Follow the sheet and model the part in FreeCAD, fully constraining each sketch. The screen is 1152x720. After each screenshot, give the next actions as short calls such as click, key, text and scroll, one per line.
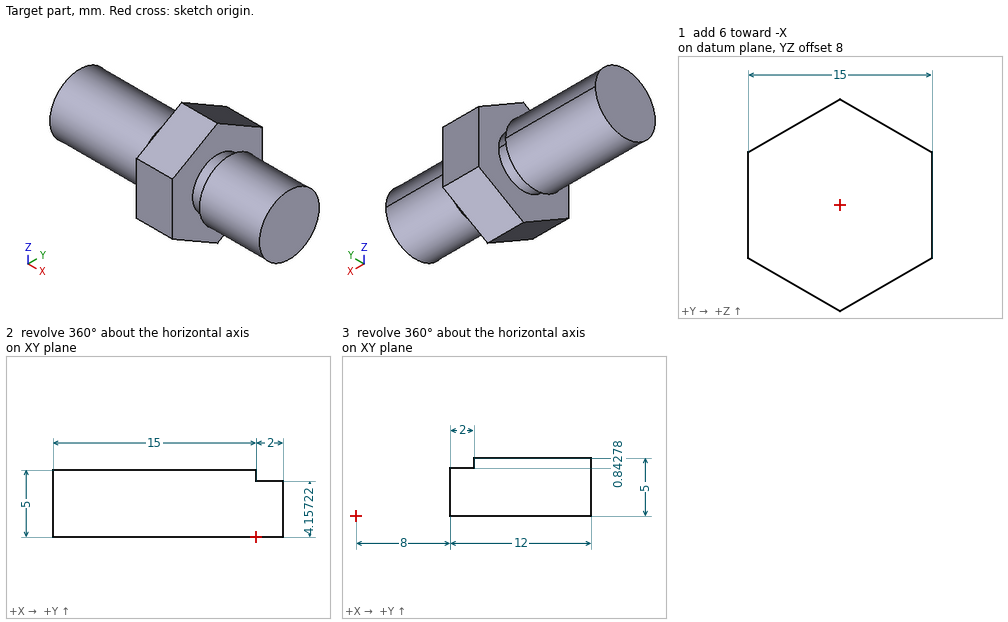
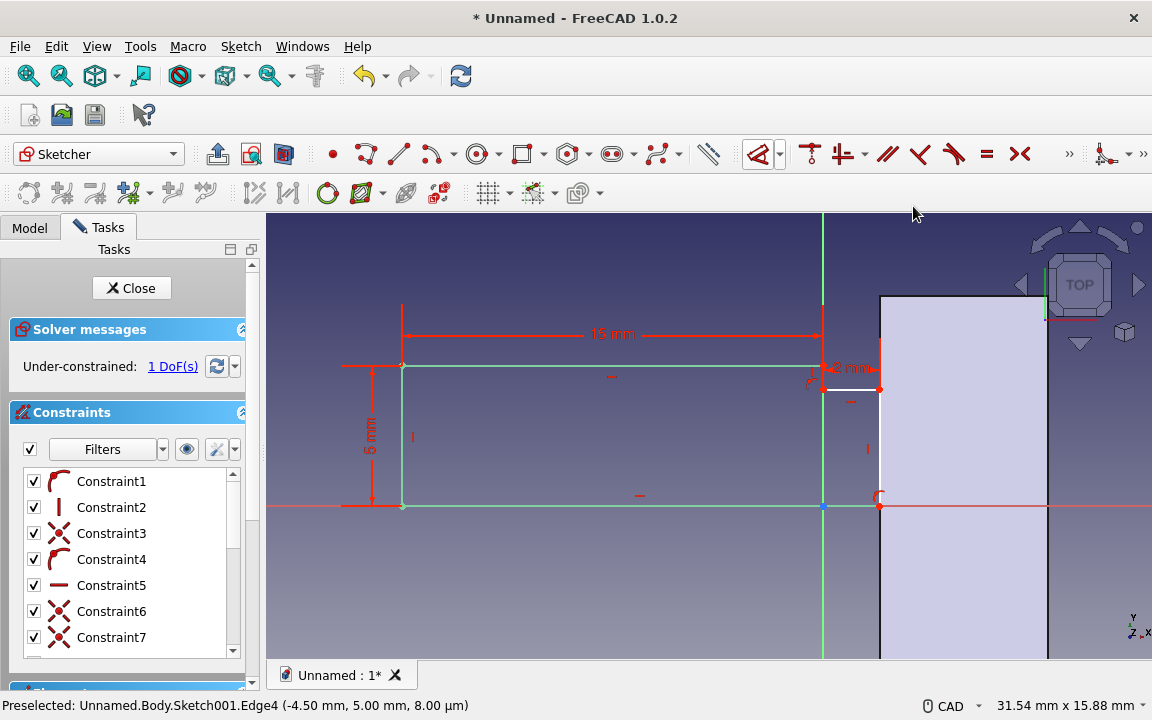
click(880, 471)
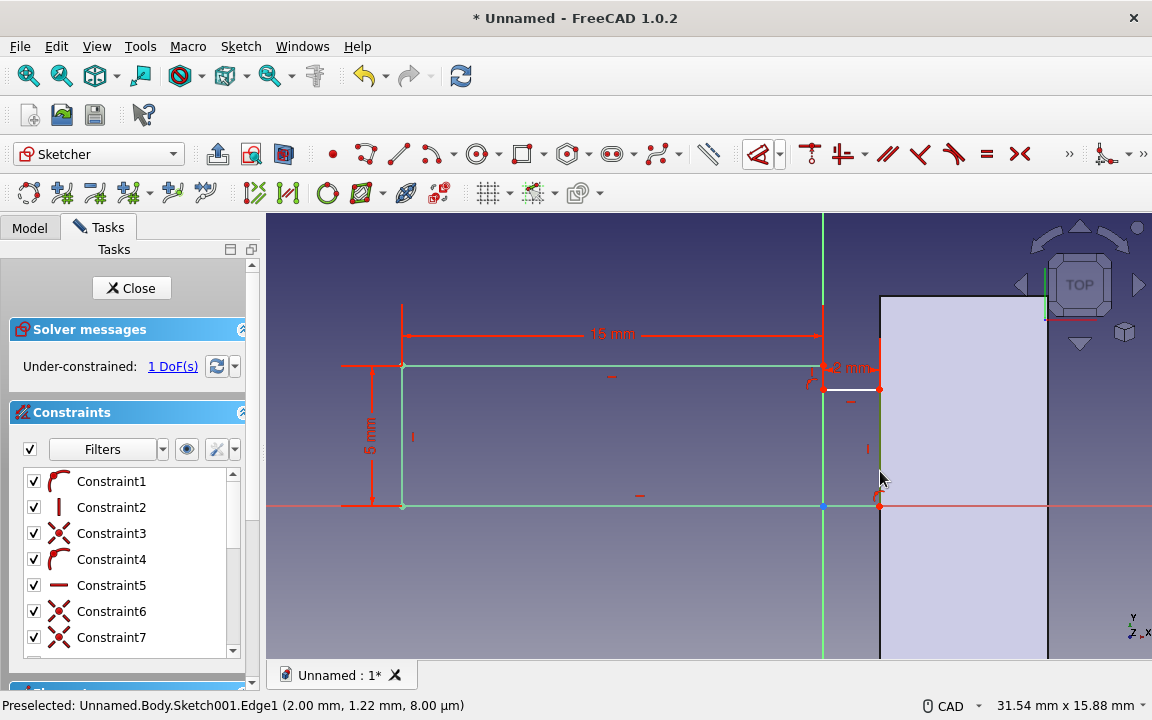
key(i)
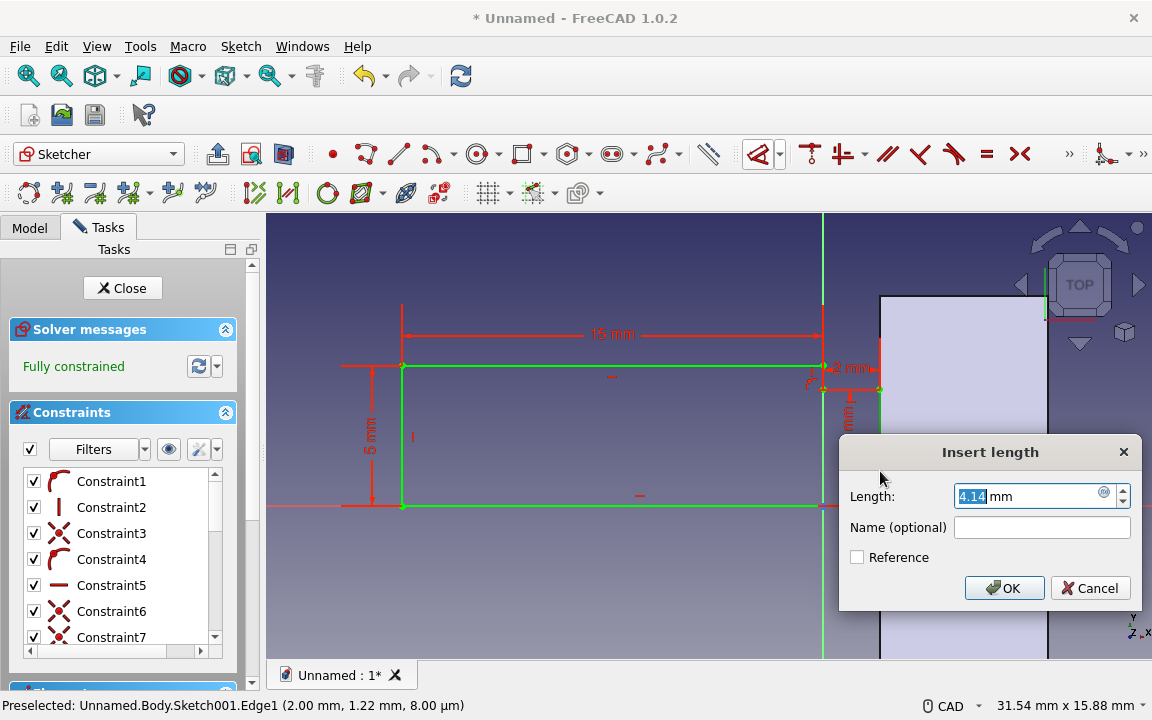
text(4.15722)
key(Return)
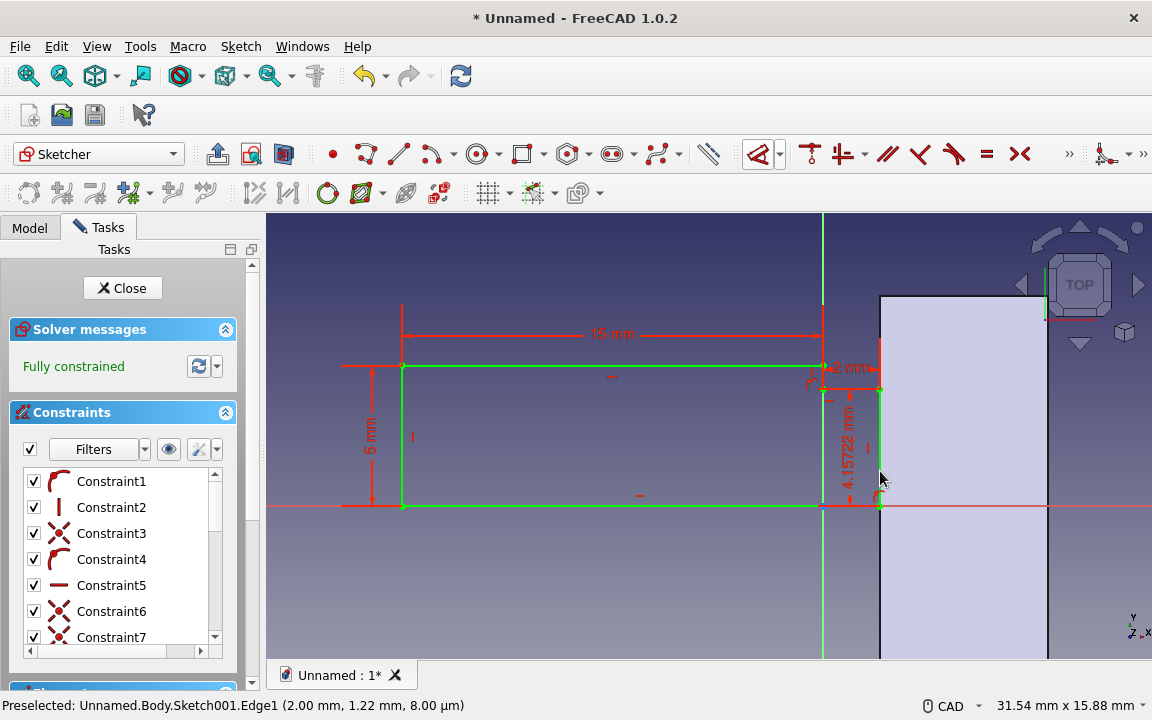
click(123, 288)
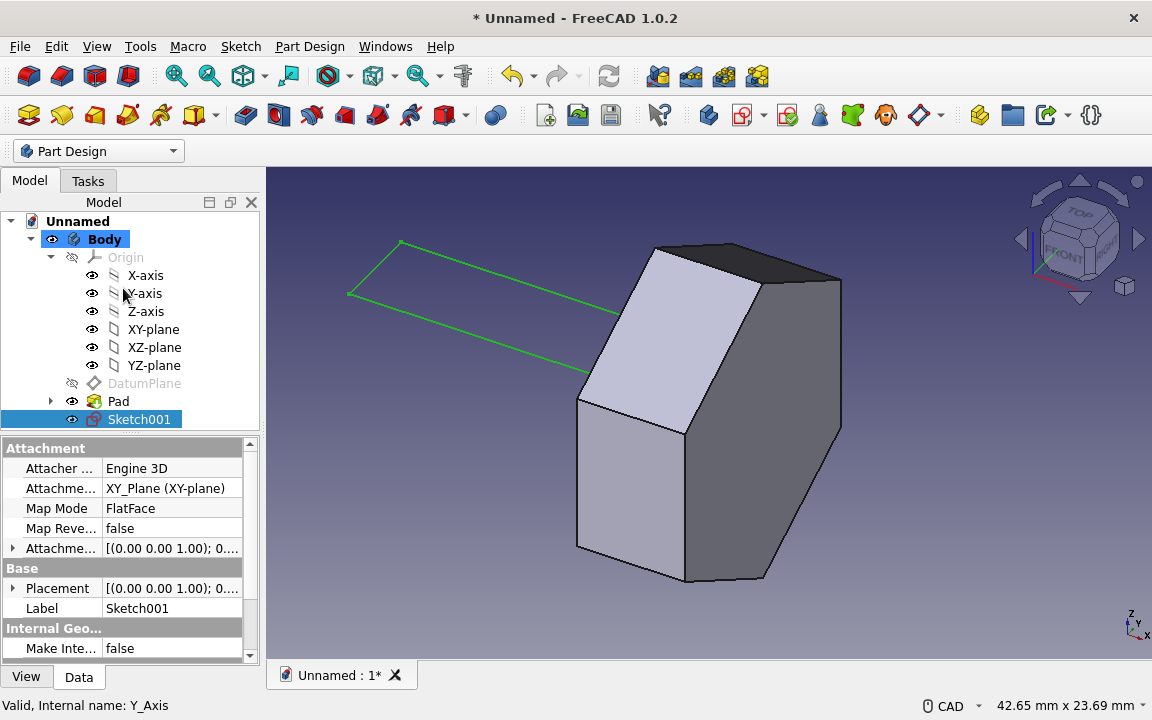
click(62, 116)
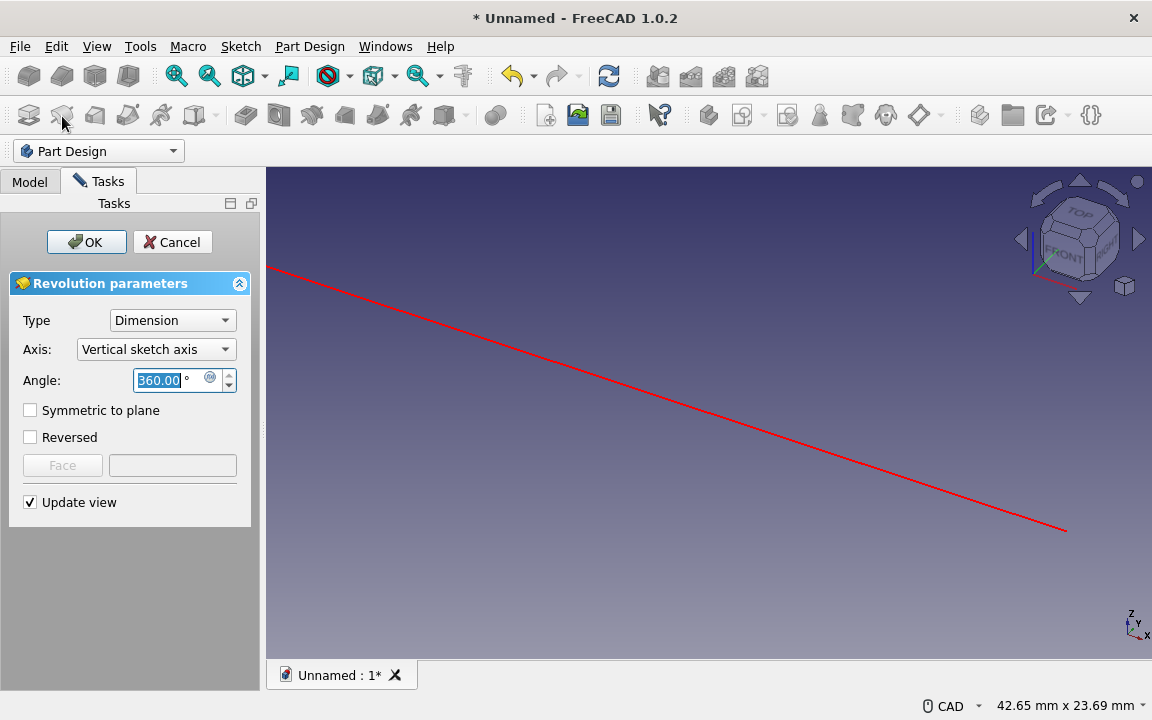
click(157, 350)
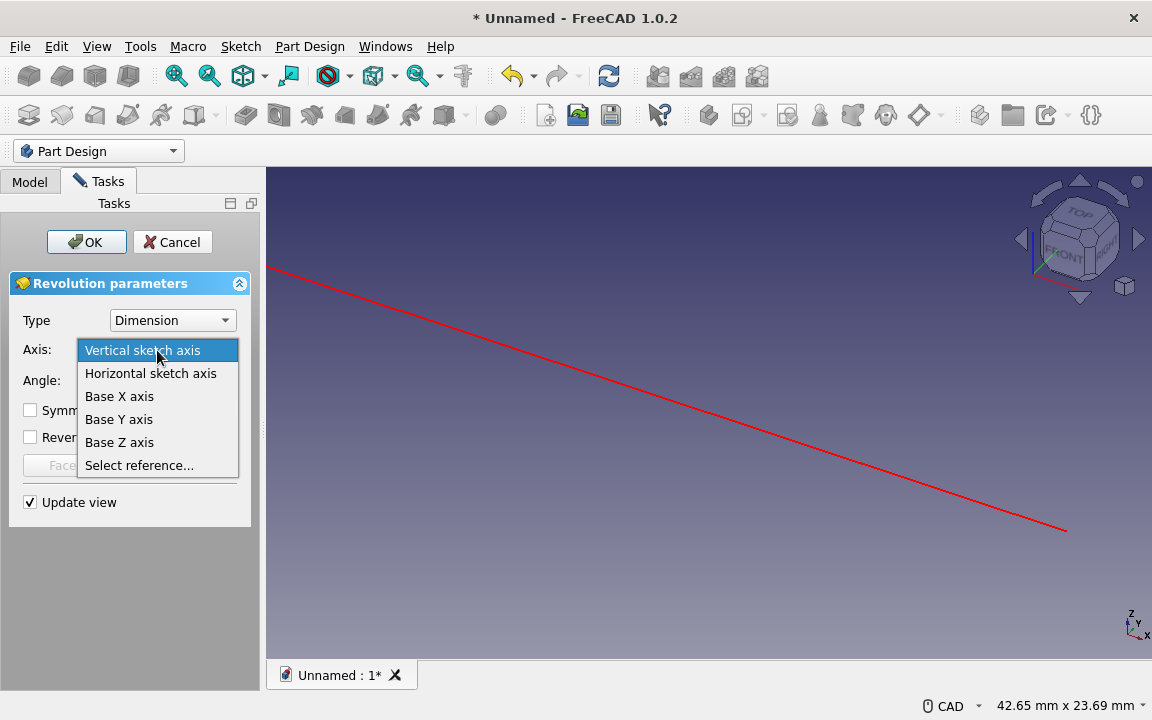
click(156, 374)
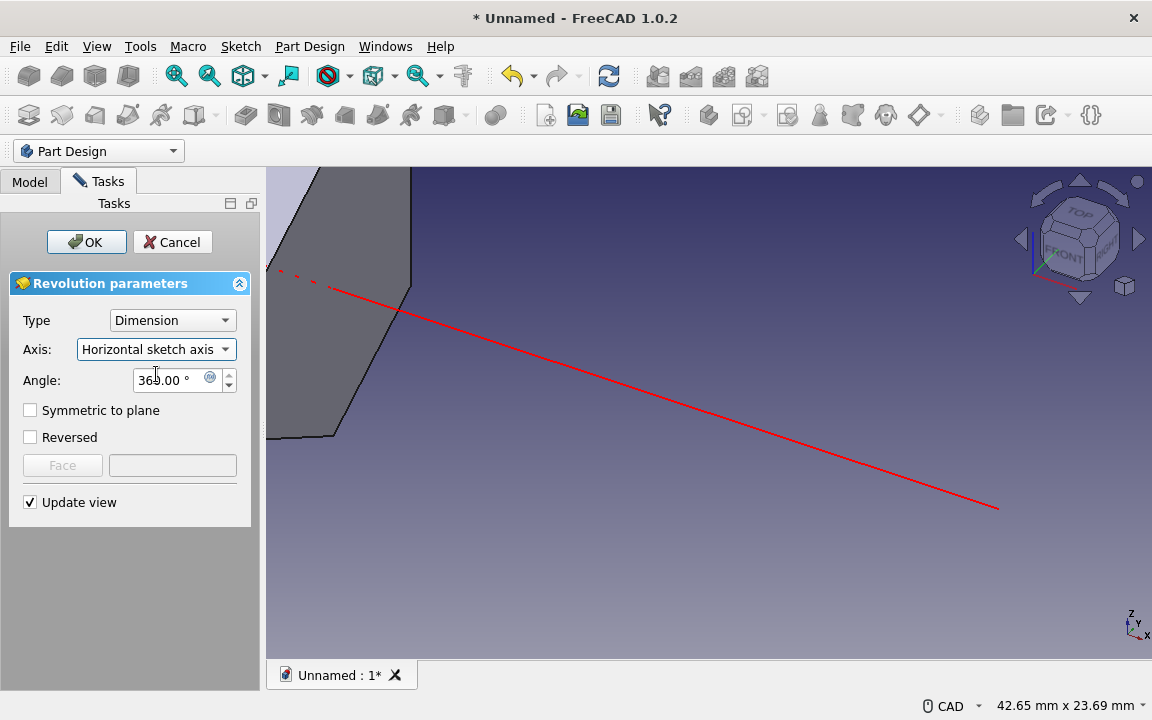
click(87, 242)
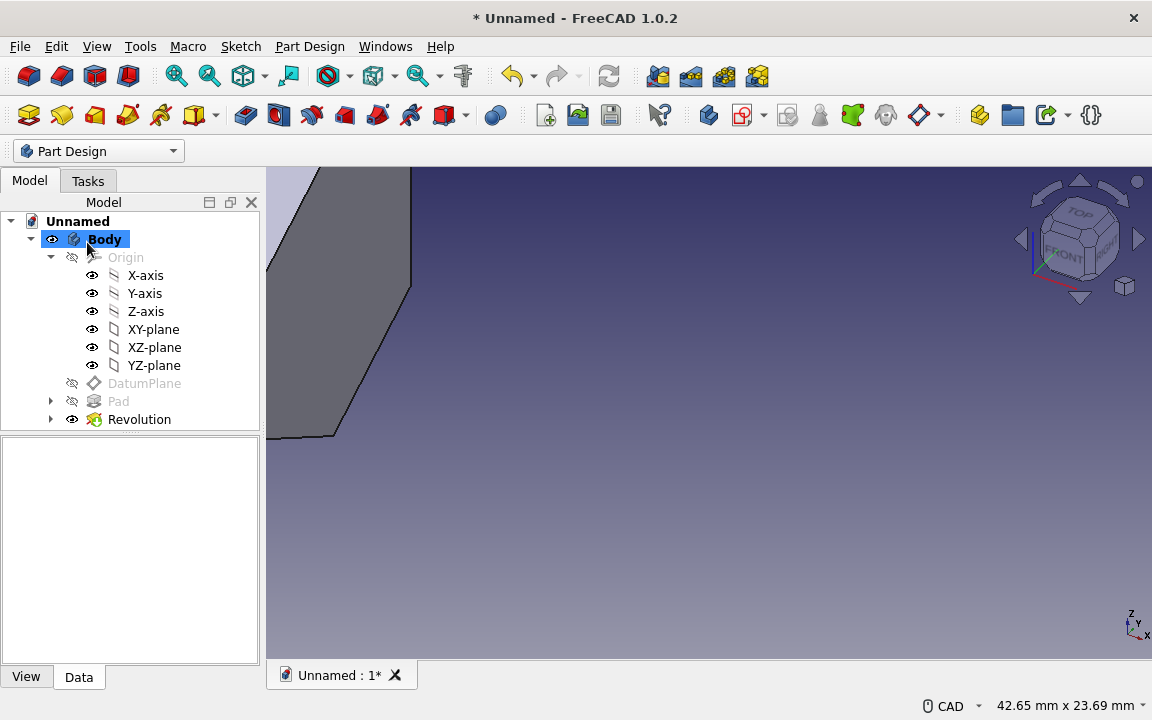
click(177, 76)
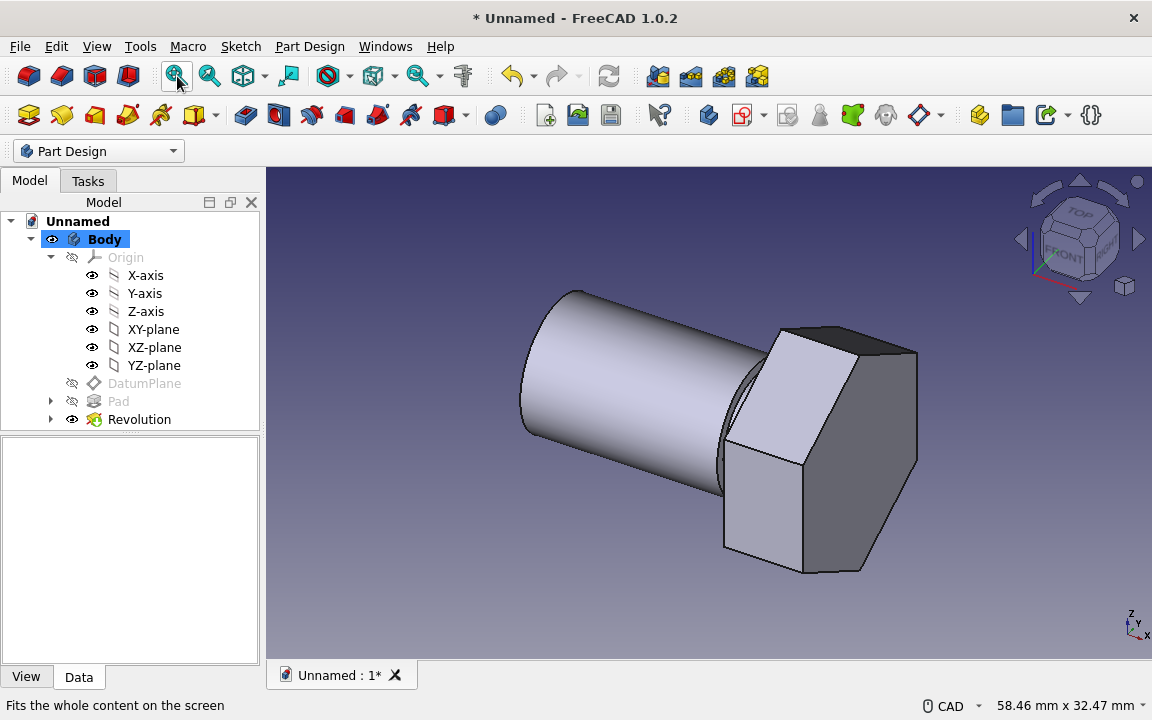
click(742, 116)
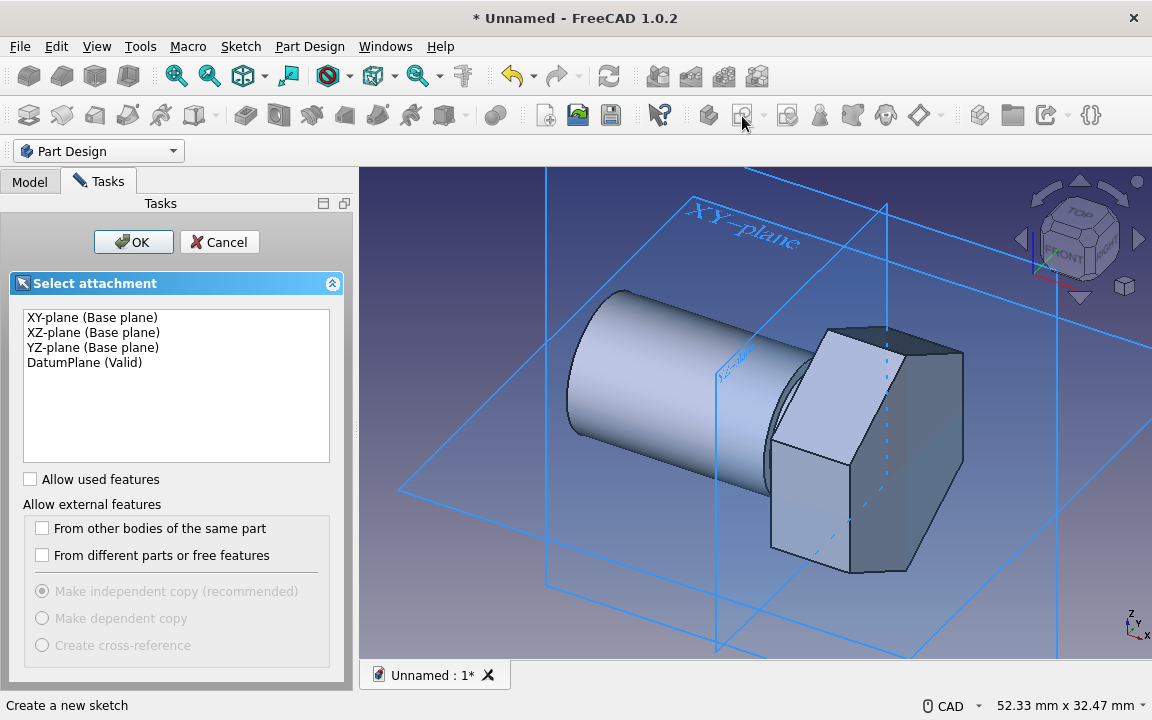
click(84, 318)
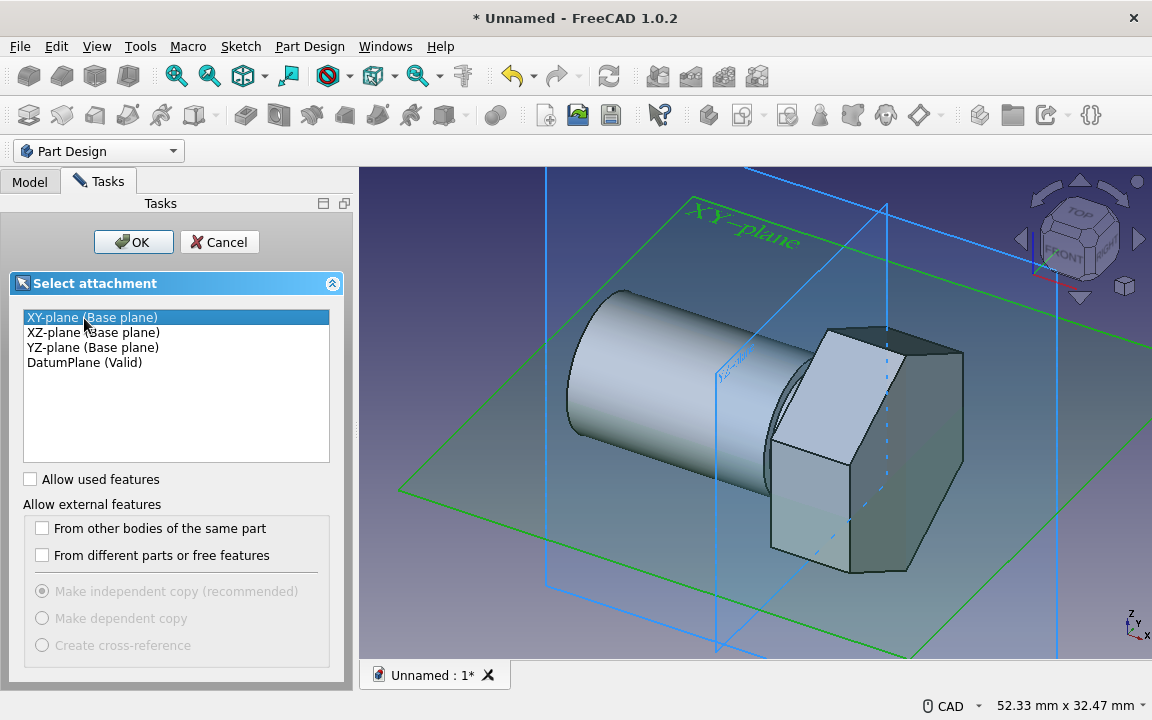
click(134, 242)